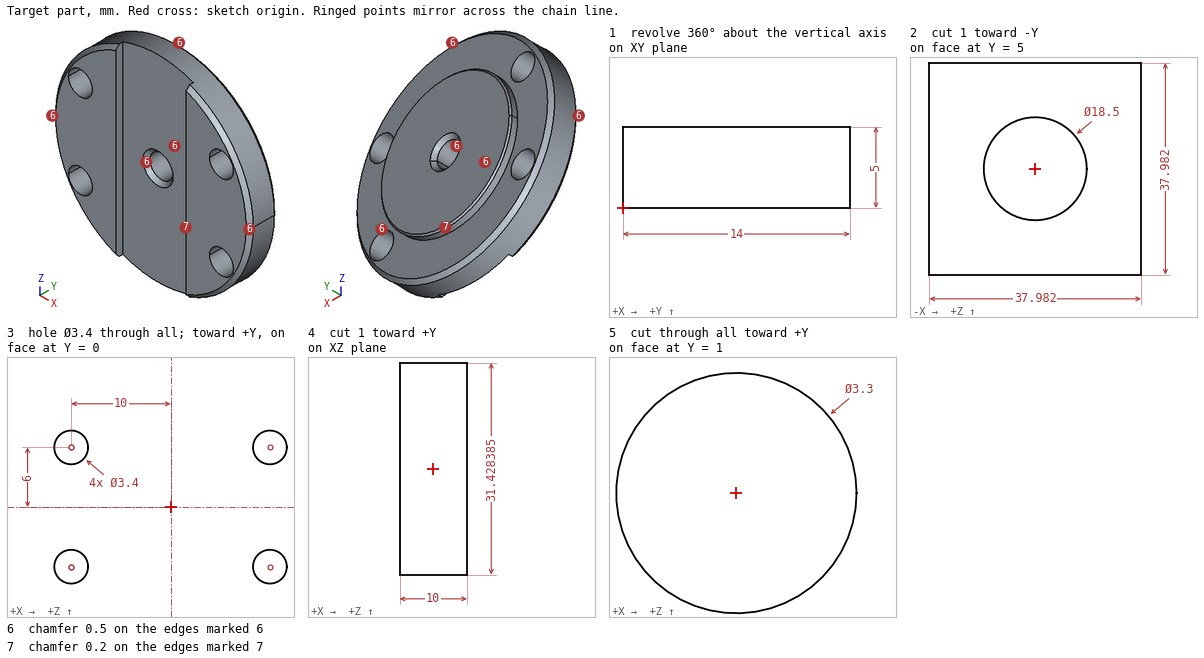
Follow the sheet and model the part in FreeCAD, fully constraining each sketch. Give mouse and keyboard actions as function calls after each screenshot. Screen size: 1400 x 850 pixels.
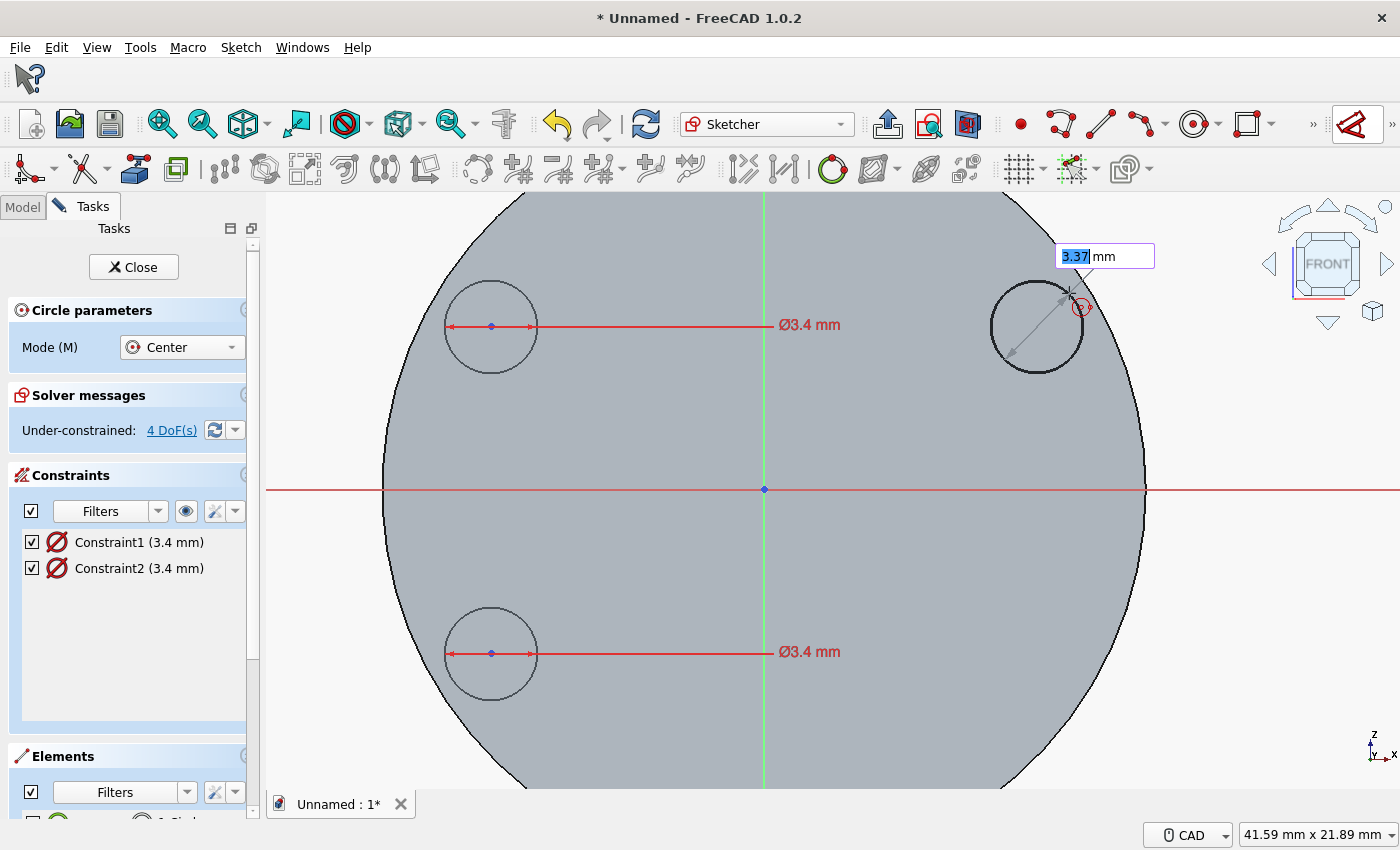
text(3.4)
key(Return)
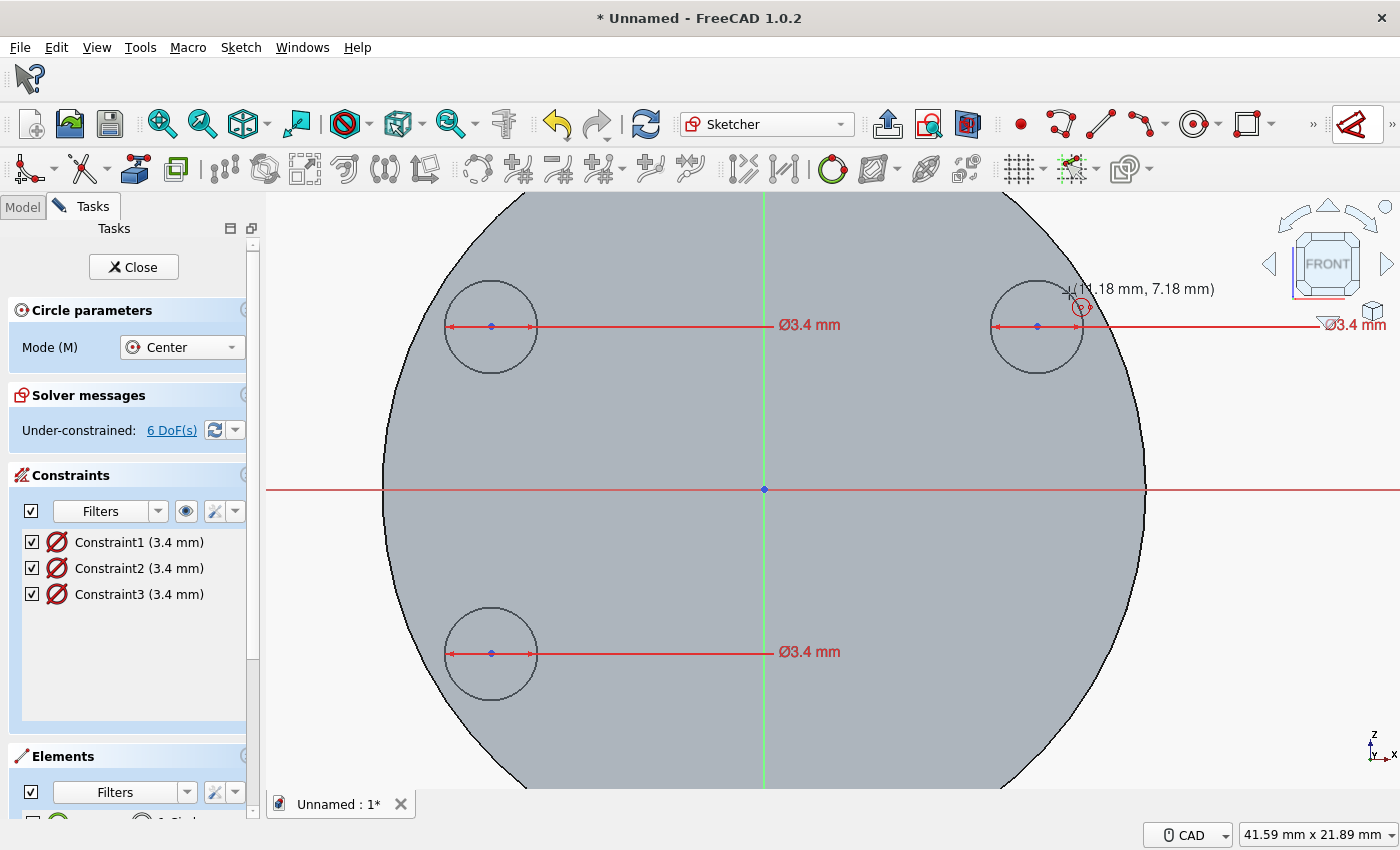
click(1037, 653)
move(1069, 621)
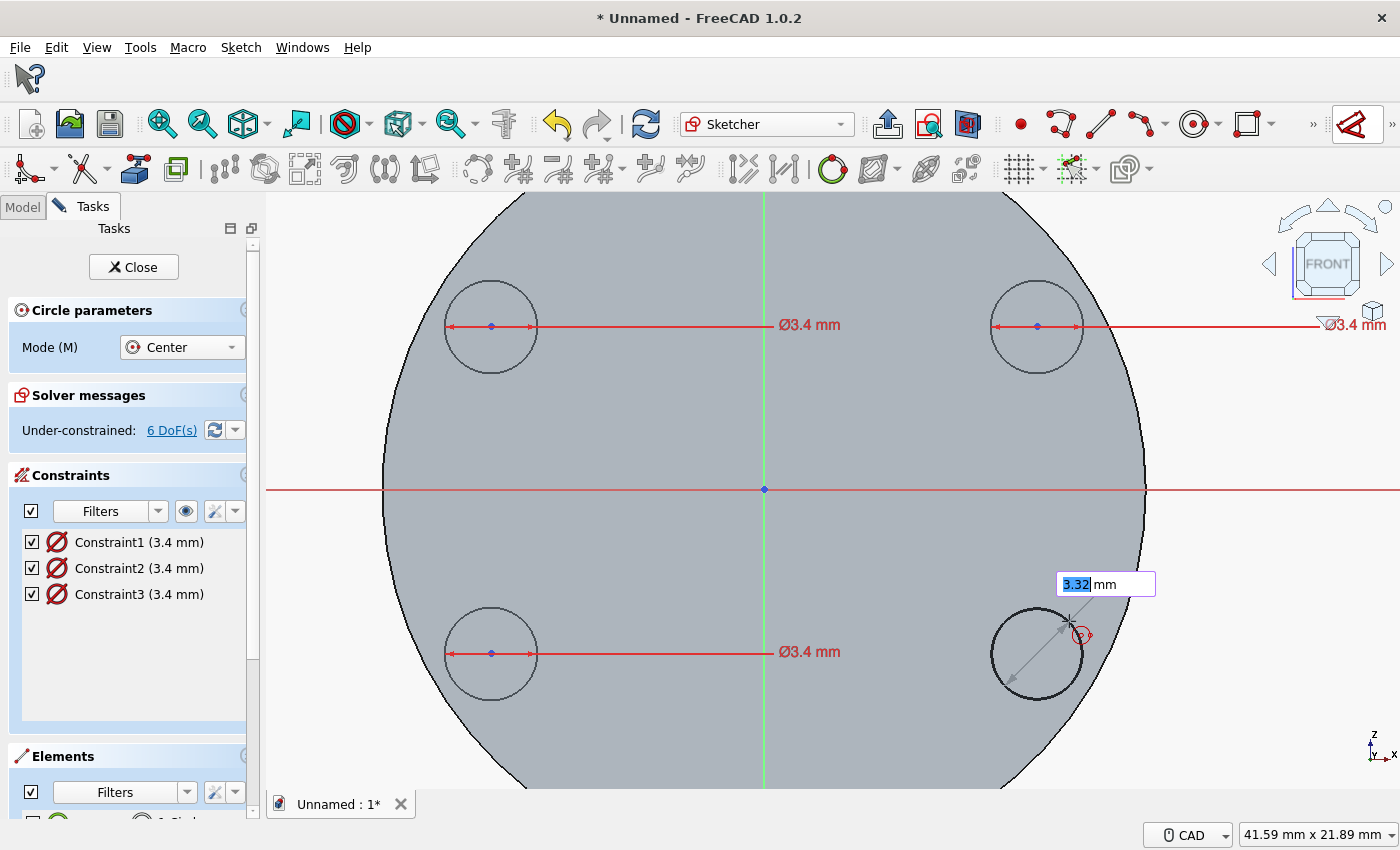
text(3.4)
key(Return)
key(Escape)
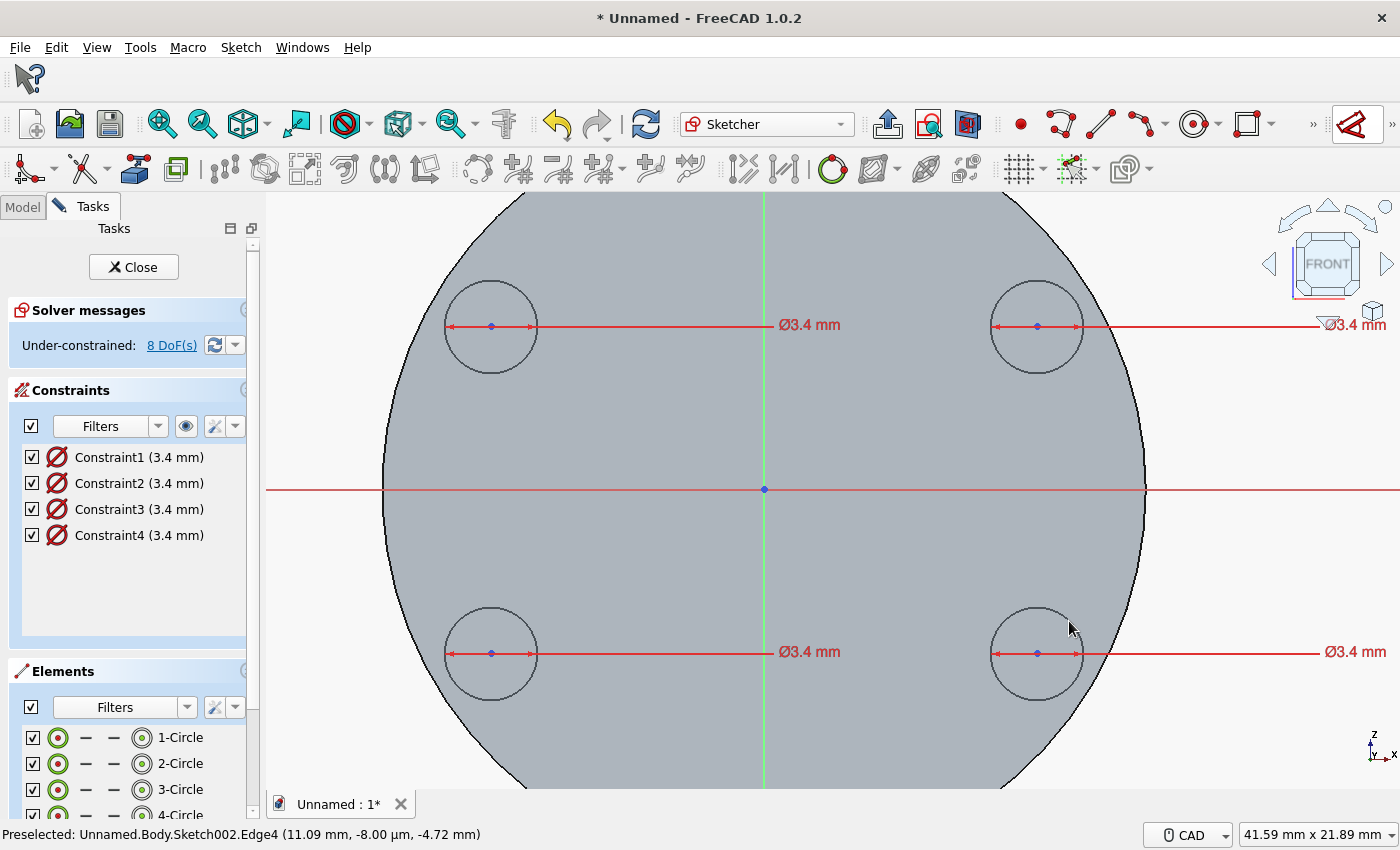
click(491, 327)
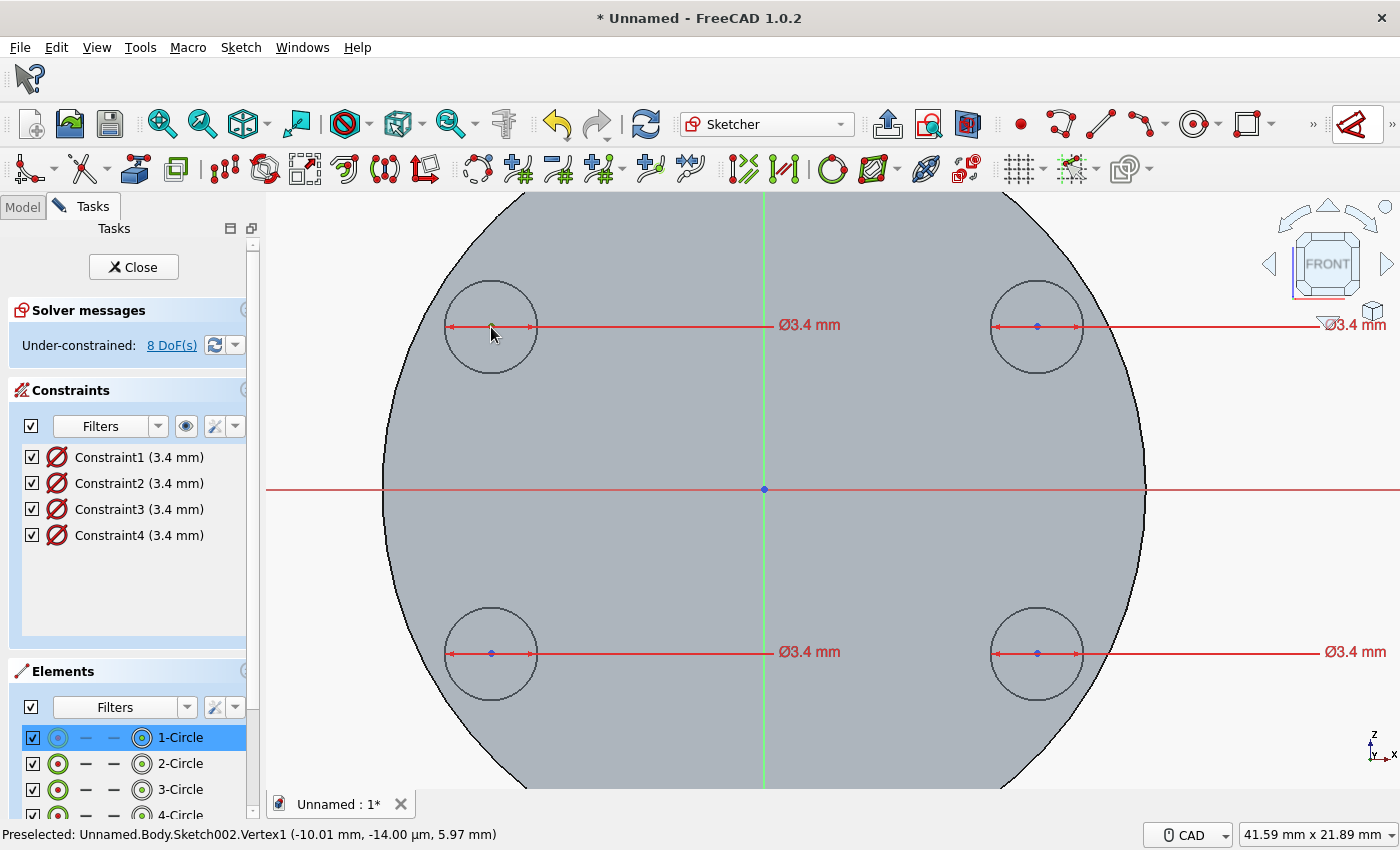
click(491, 654)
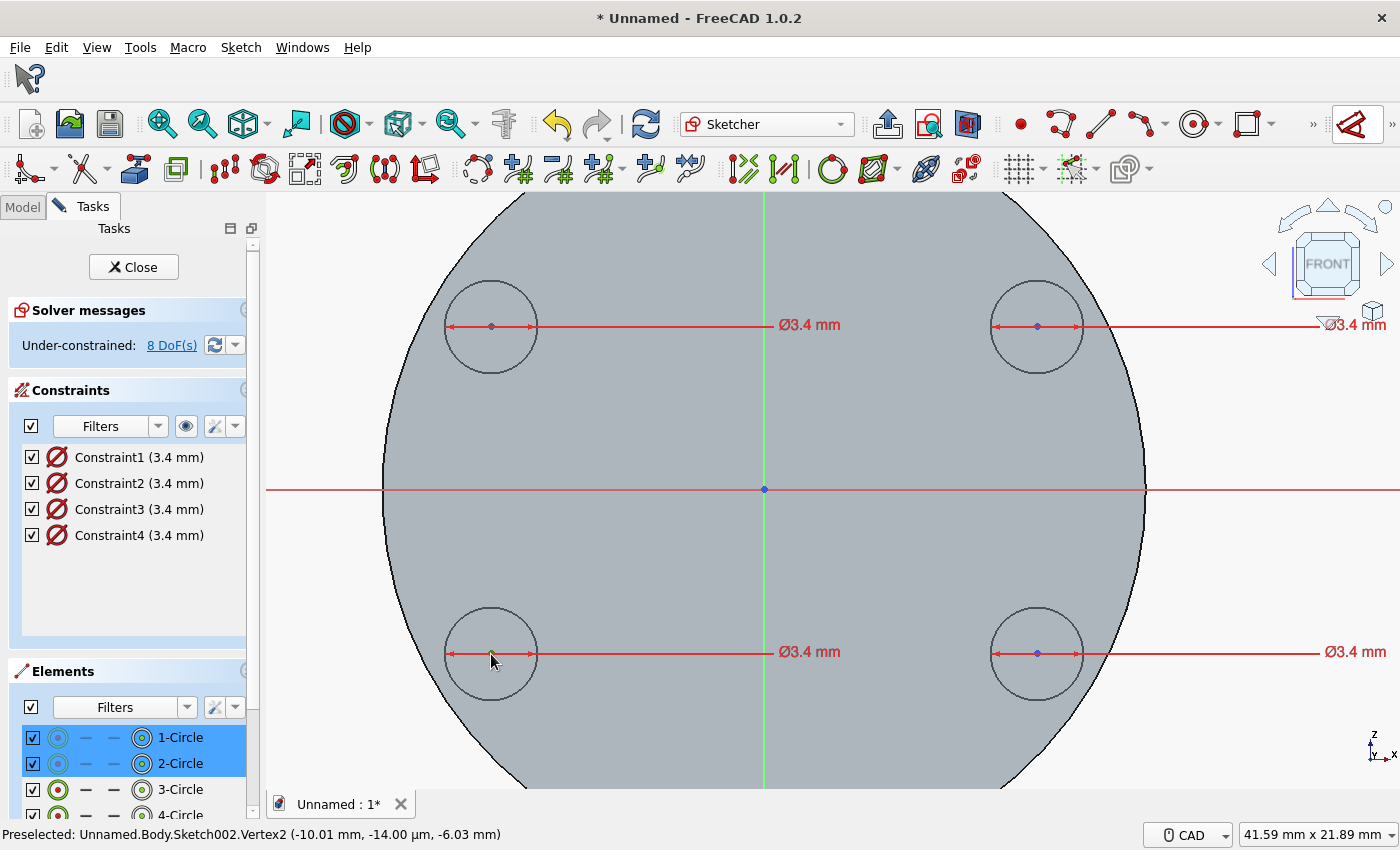
click(361, 490)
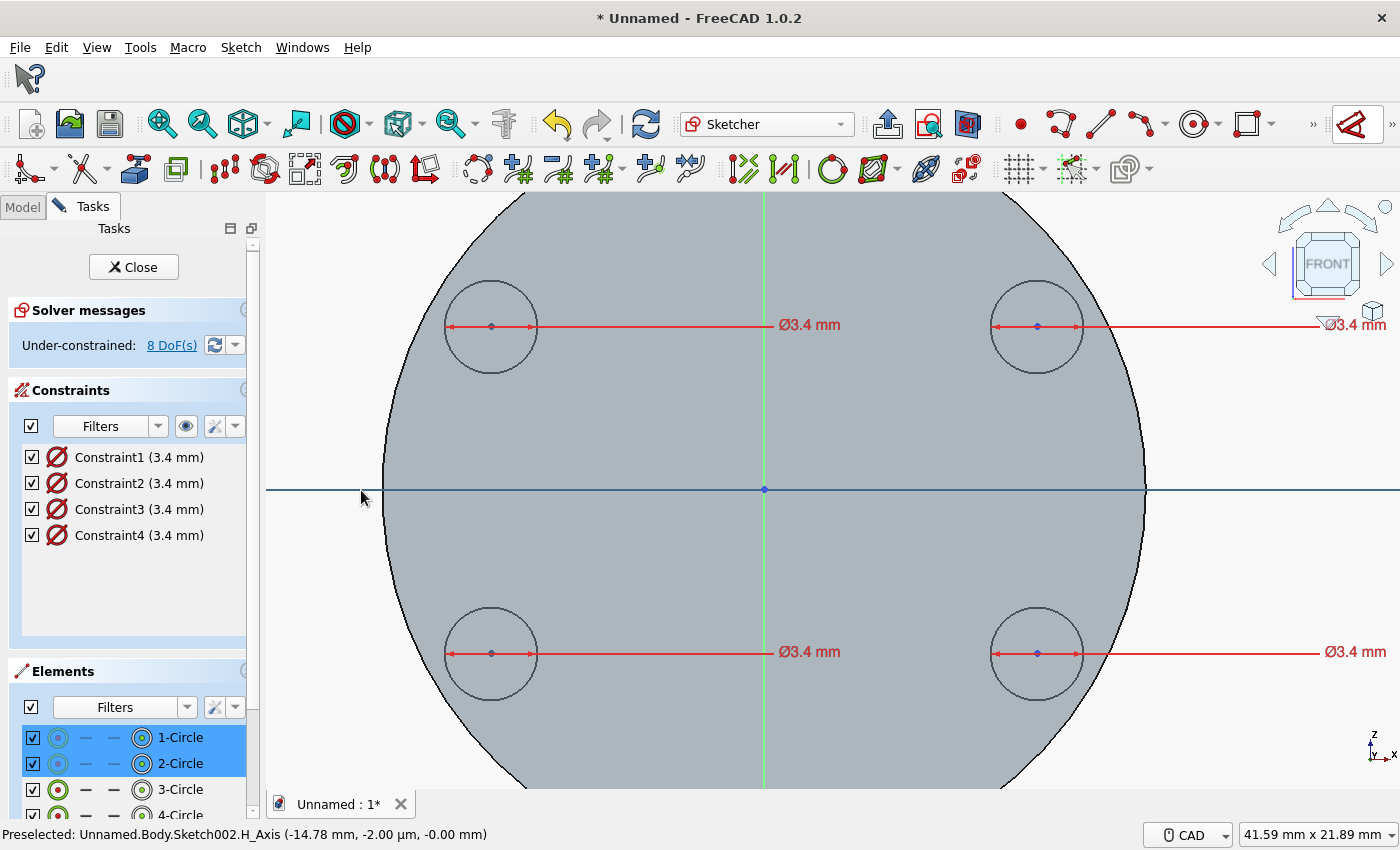
key(s)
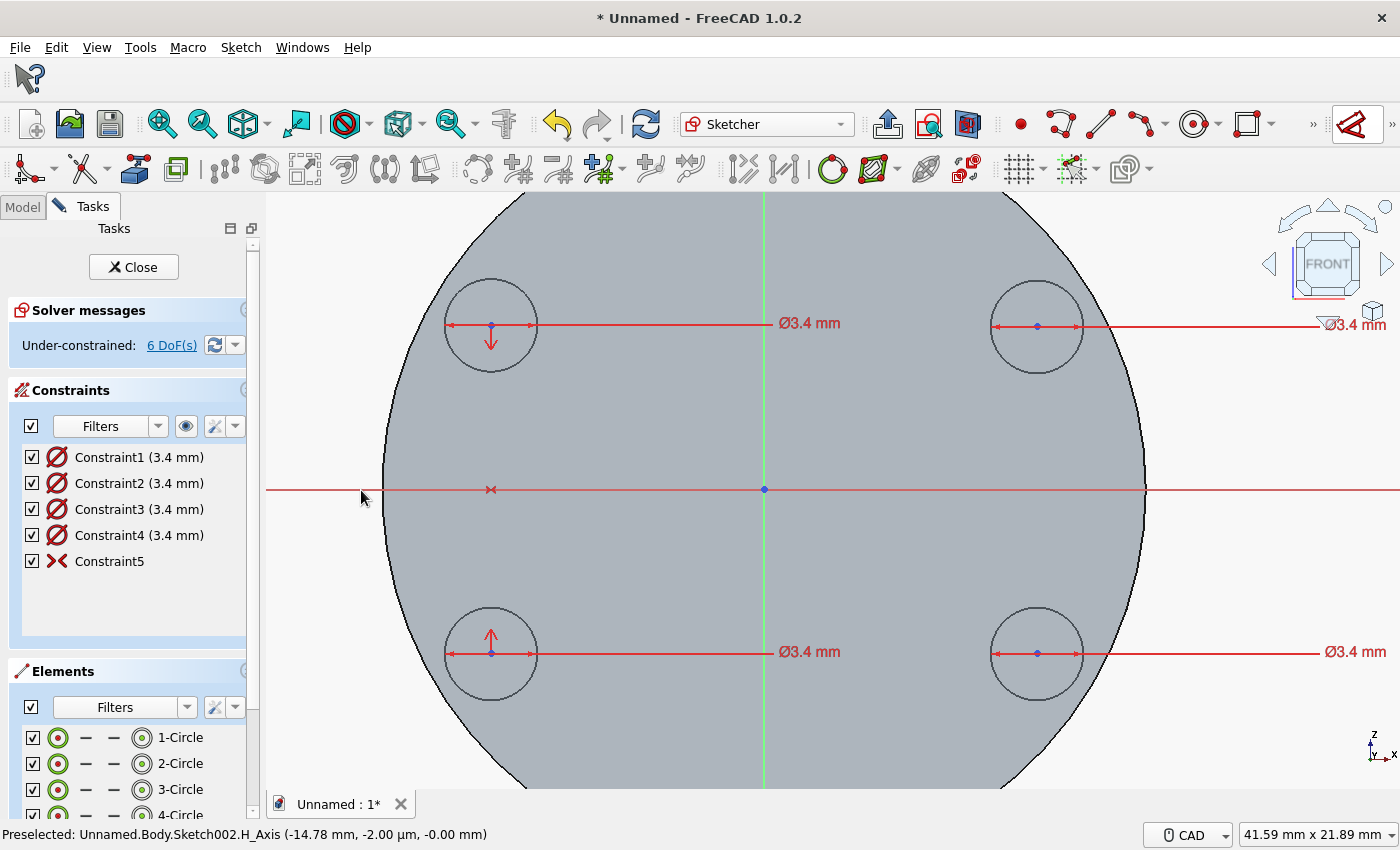
click(491, 325)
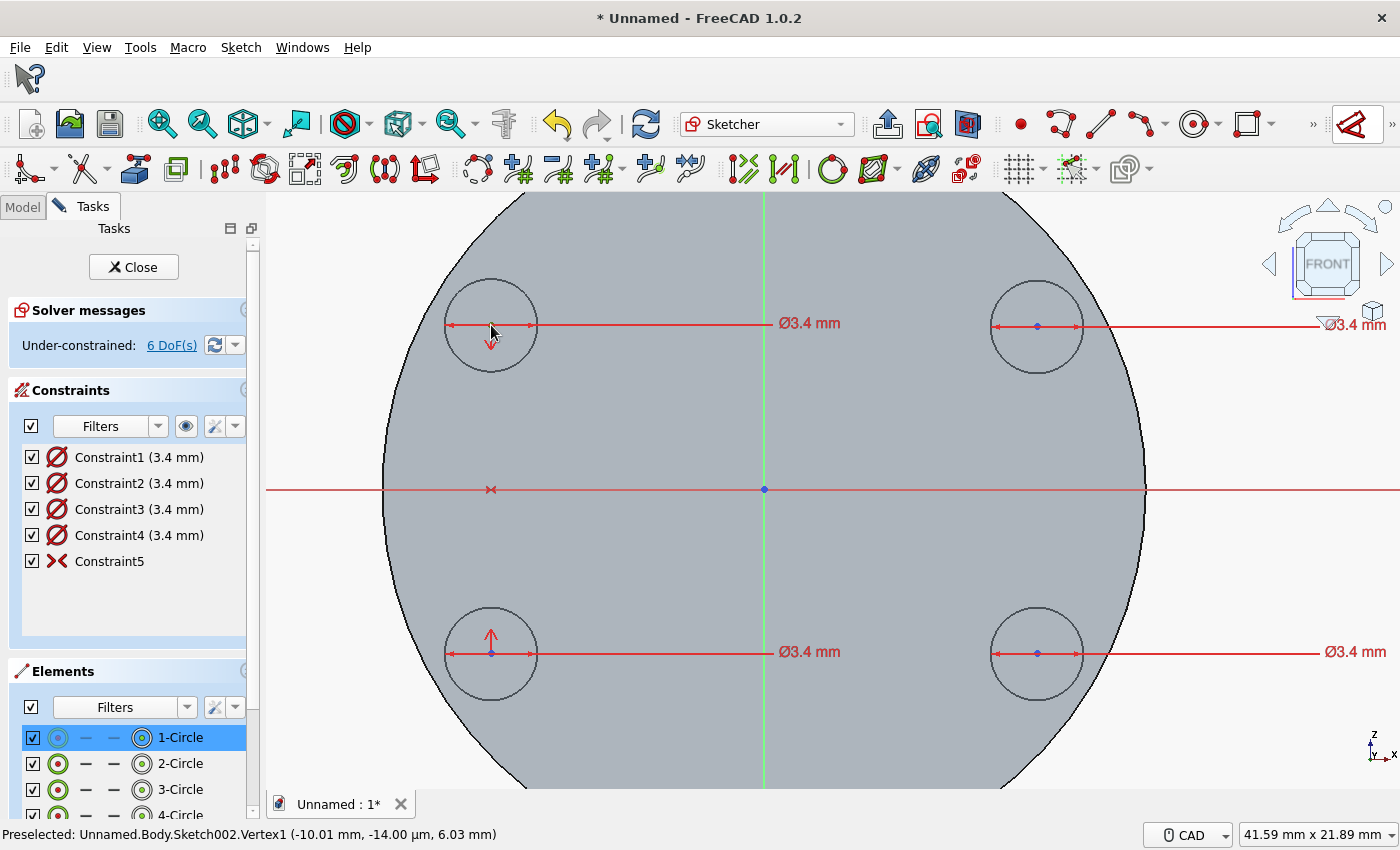
click(1037, 327)